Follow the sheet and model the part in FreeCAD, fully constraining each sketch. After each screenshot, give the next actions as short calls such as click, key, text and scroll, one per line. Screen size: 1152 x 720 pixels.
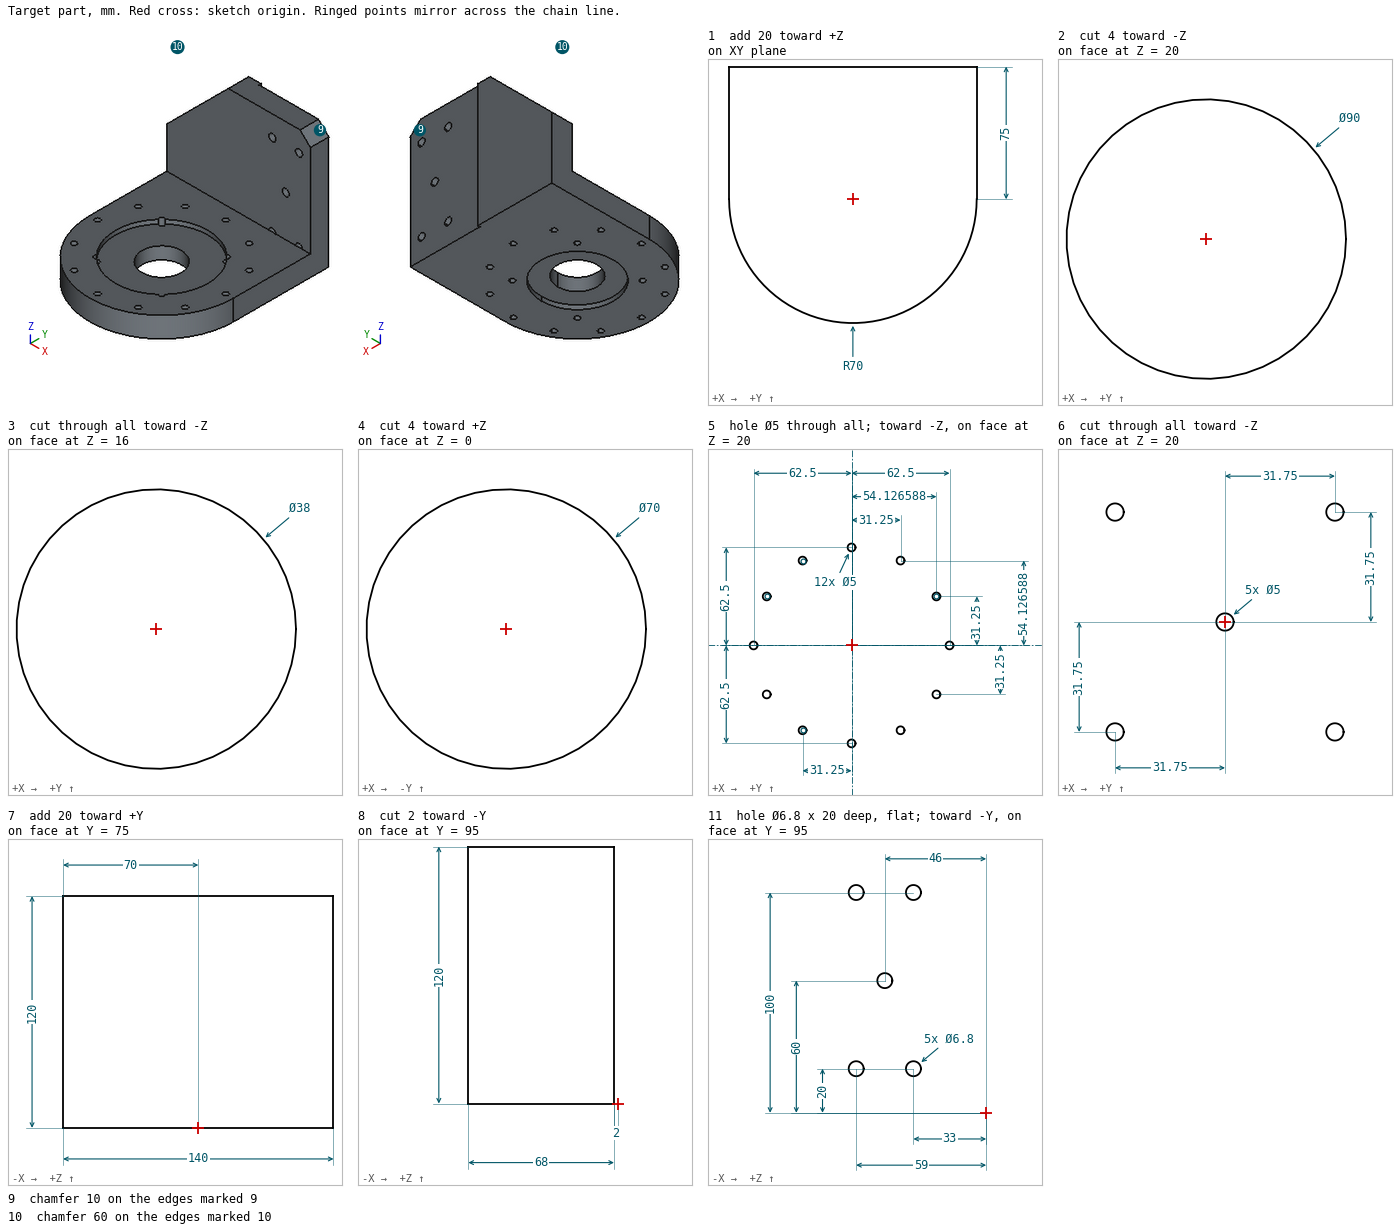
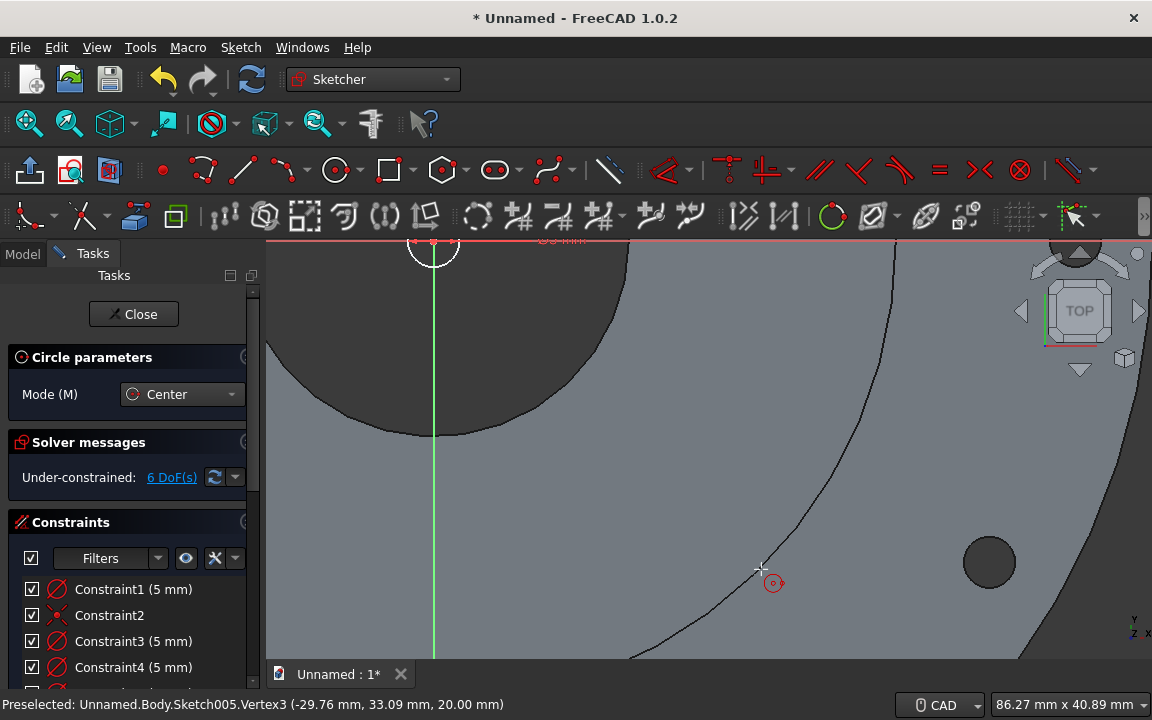
click(760, 567)
move(778, 549)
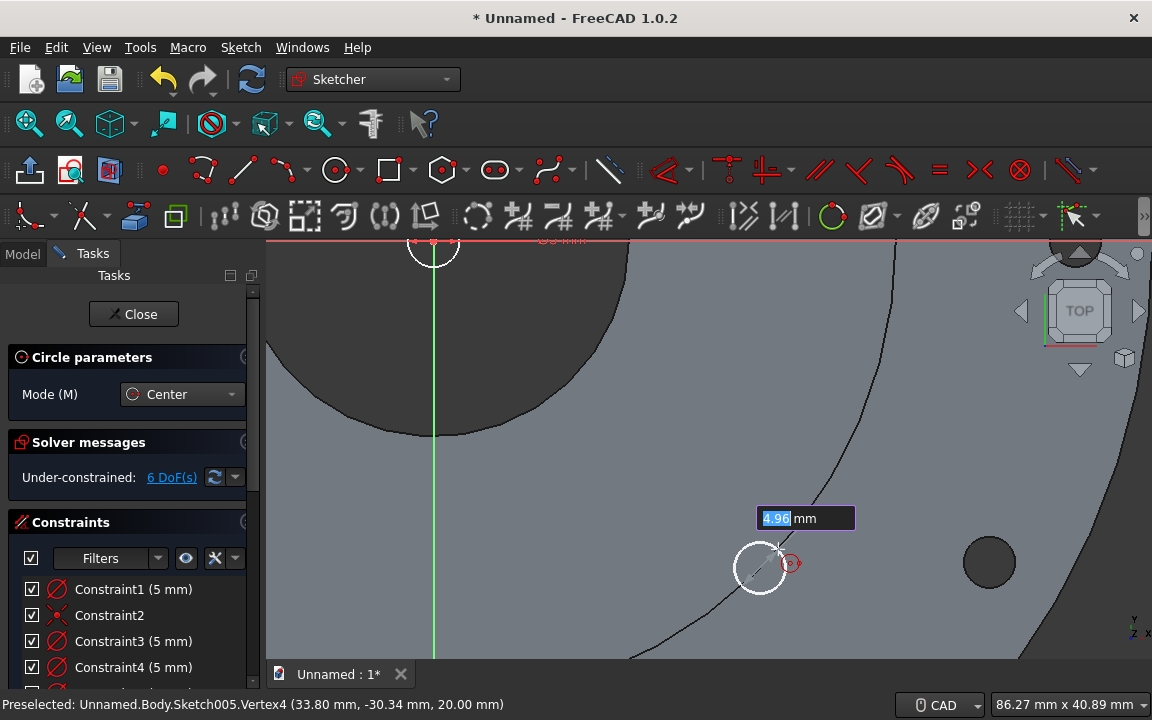
text(5)
key(Return)
key(Escape)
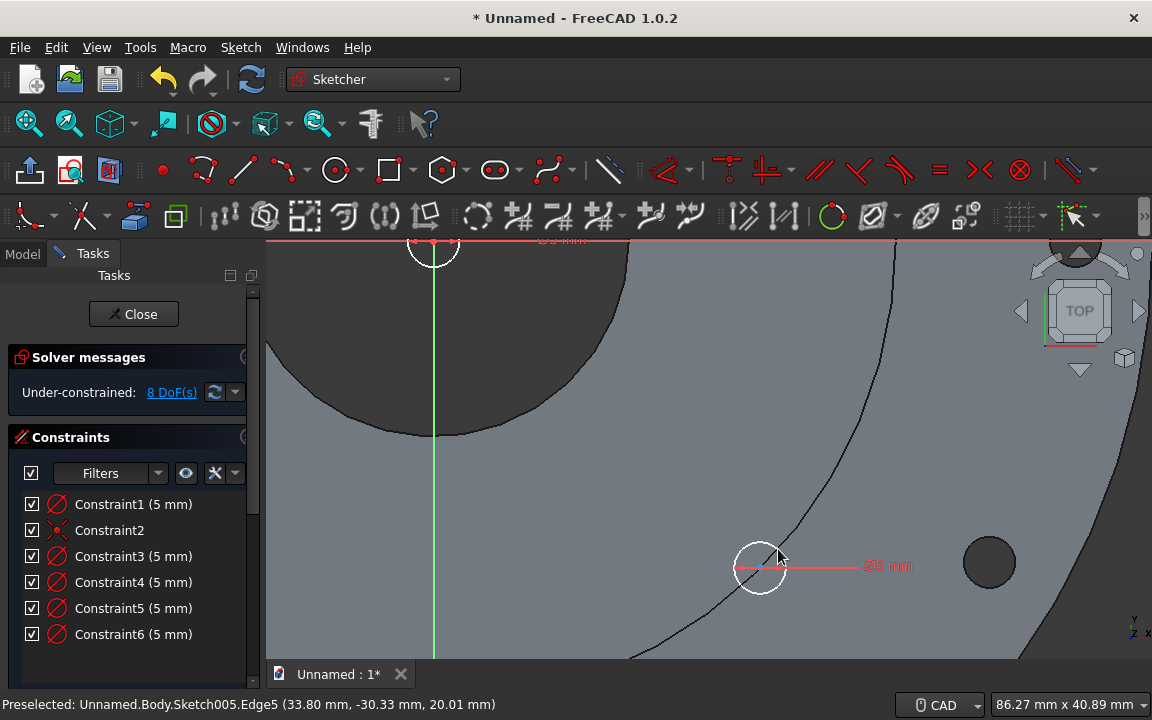
scroll(761, 570, down, 5)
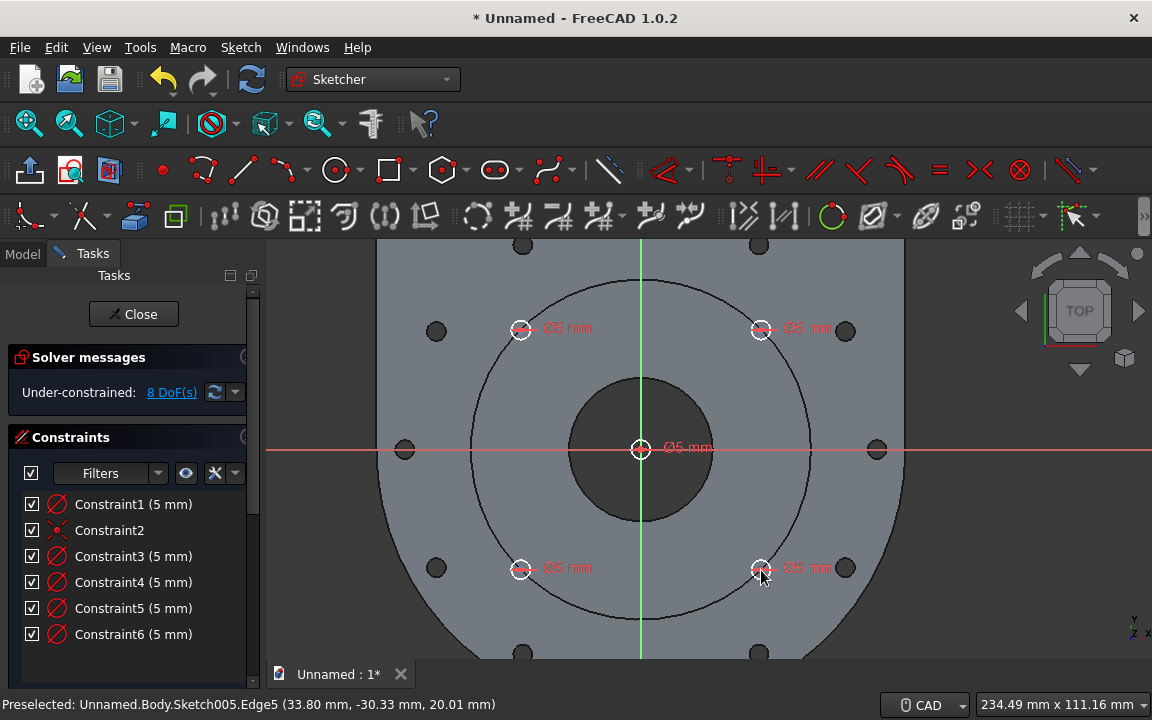
click(521, 570)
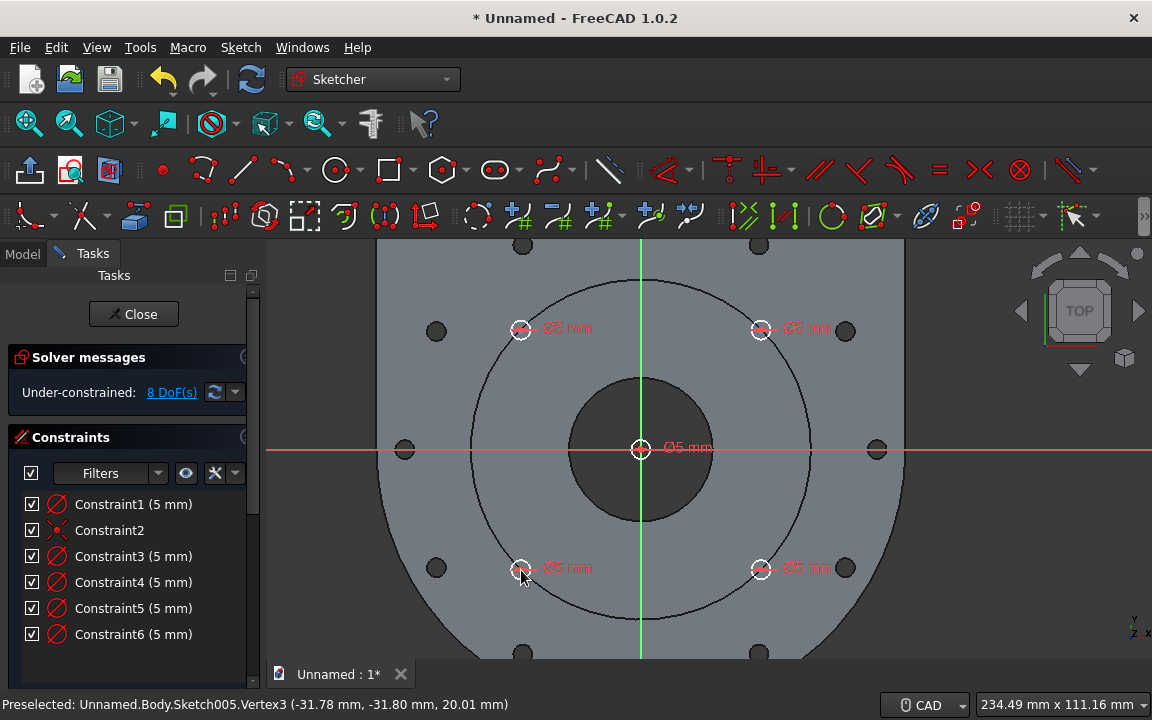
click(521, 330)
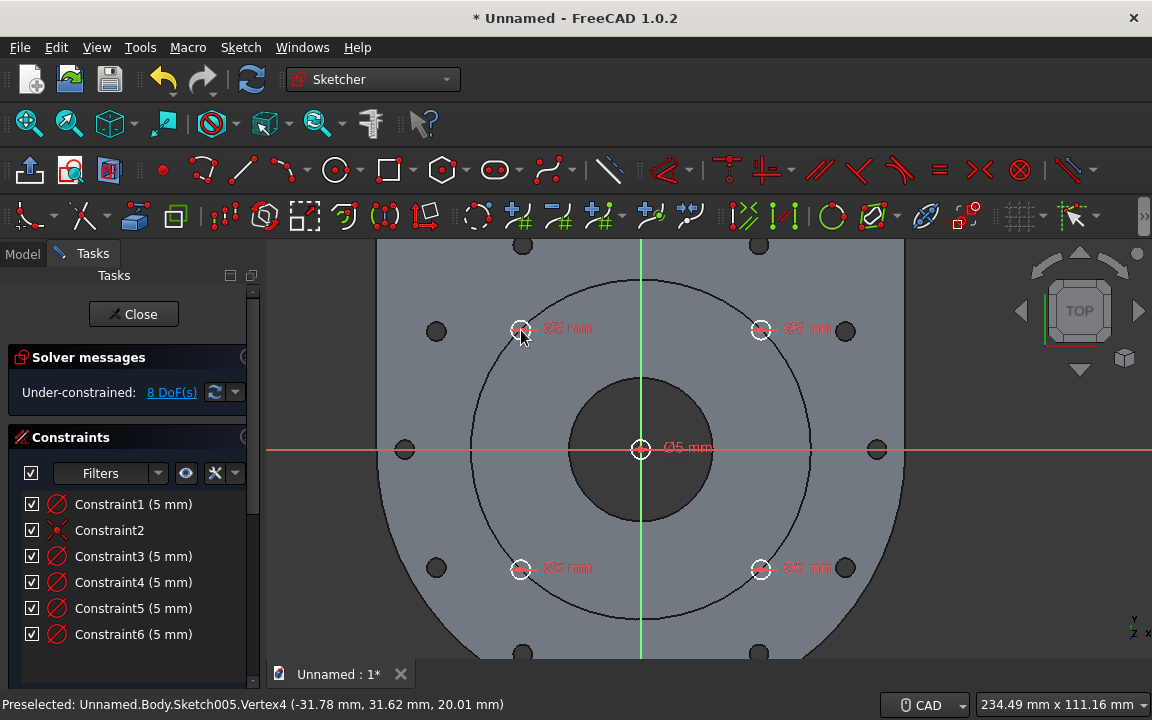
key(v)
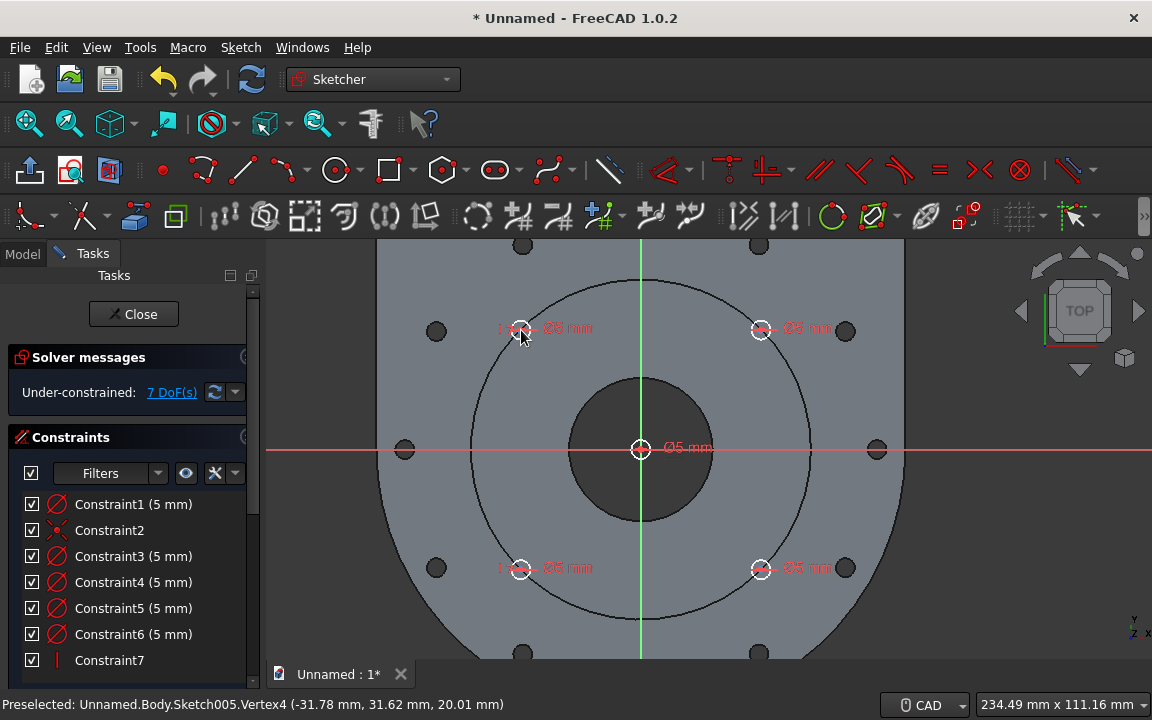
click(761, 330)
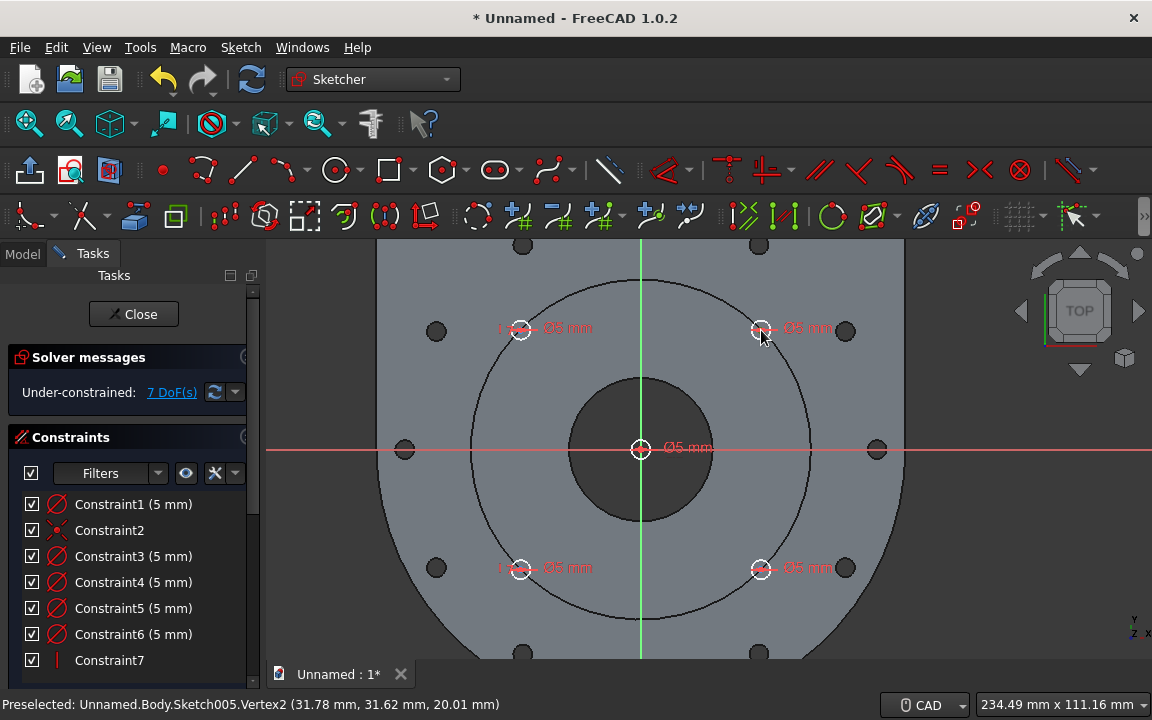
click(521, 330)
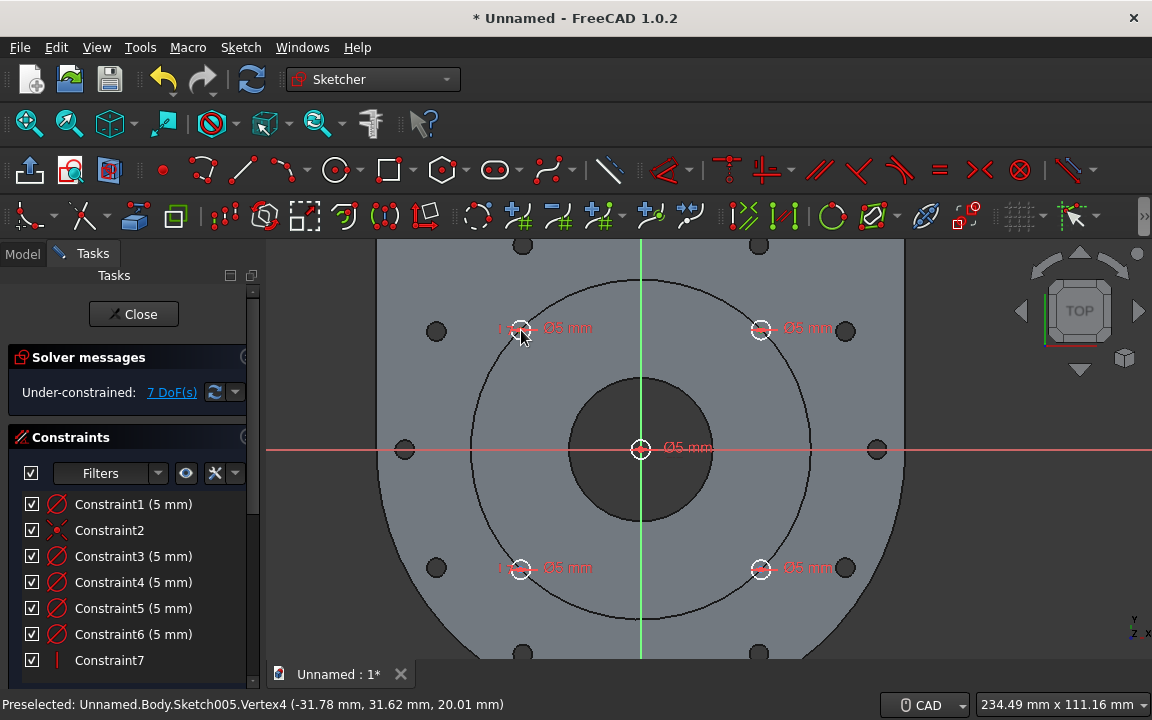
click(794, 170)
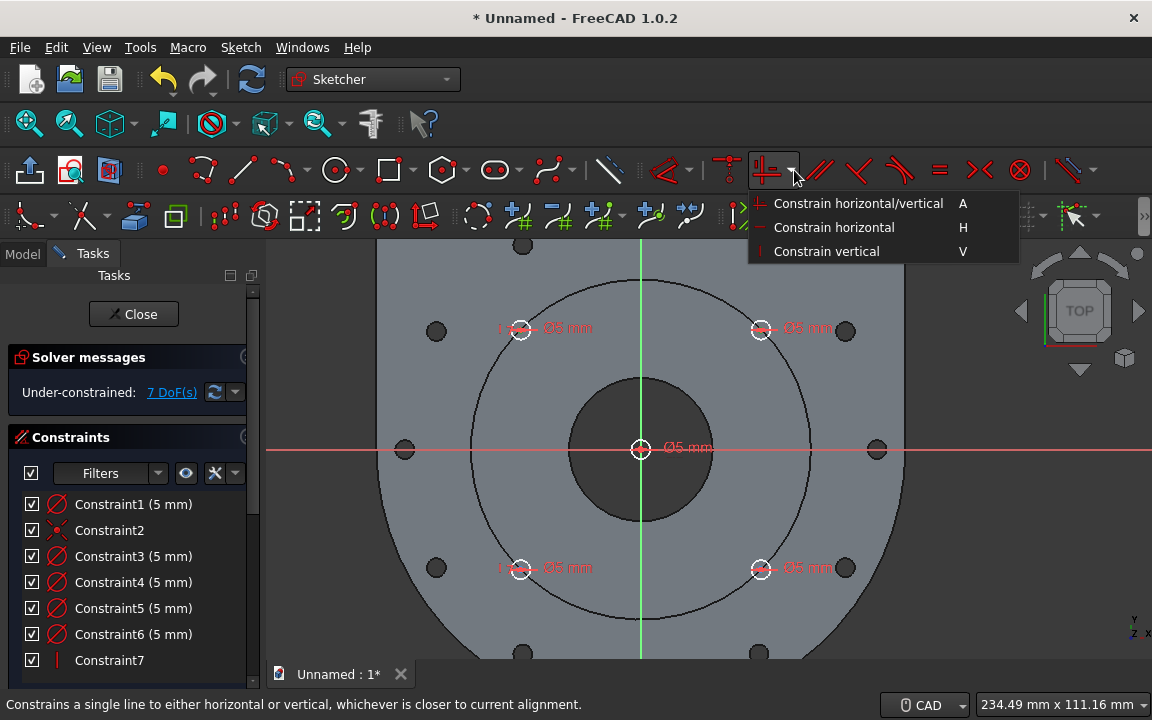
click(884, 227)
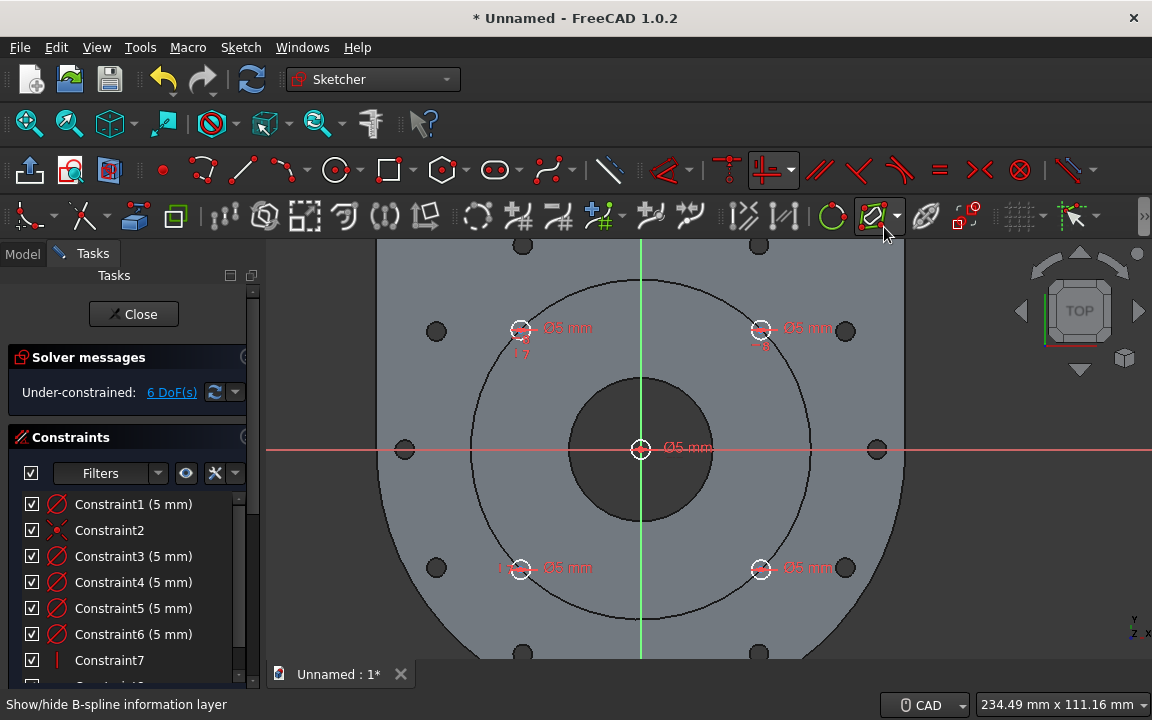
click(761, 330)